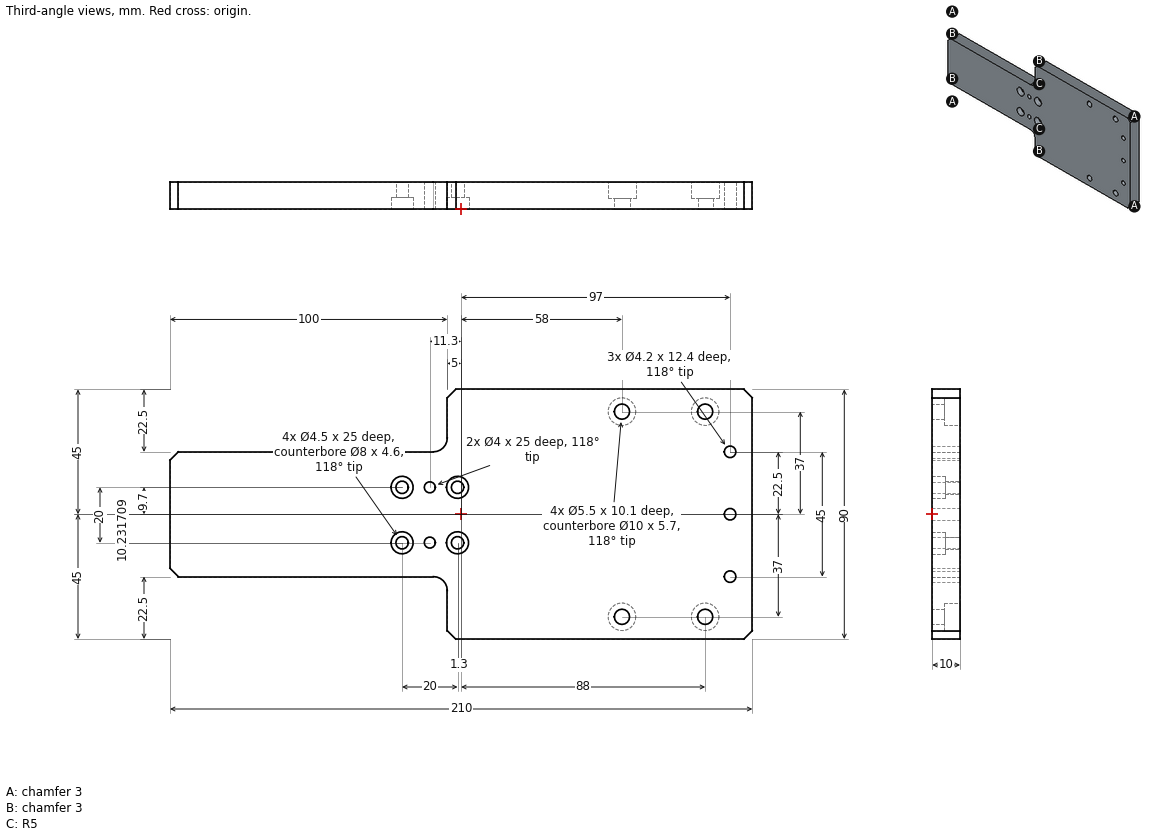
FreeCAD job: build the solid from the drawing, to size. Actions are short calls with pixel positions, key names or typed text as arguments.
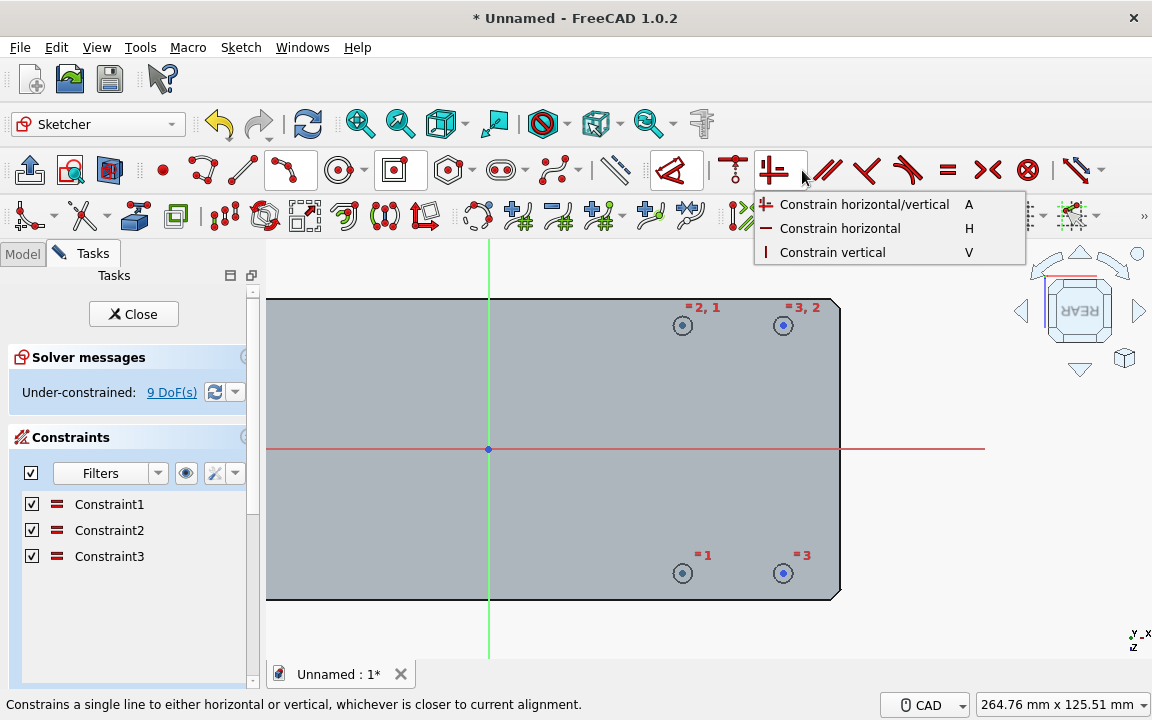
click(890, 252)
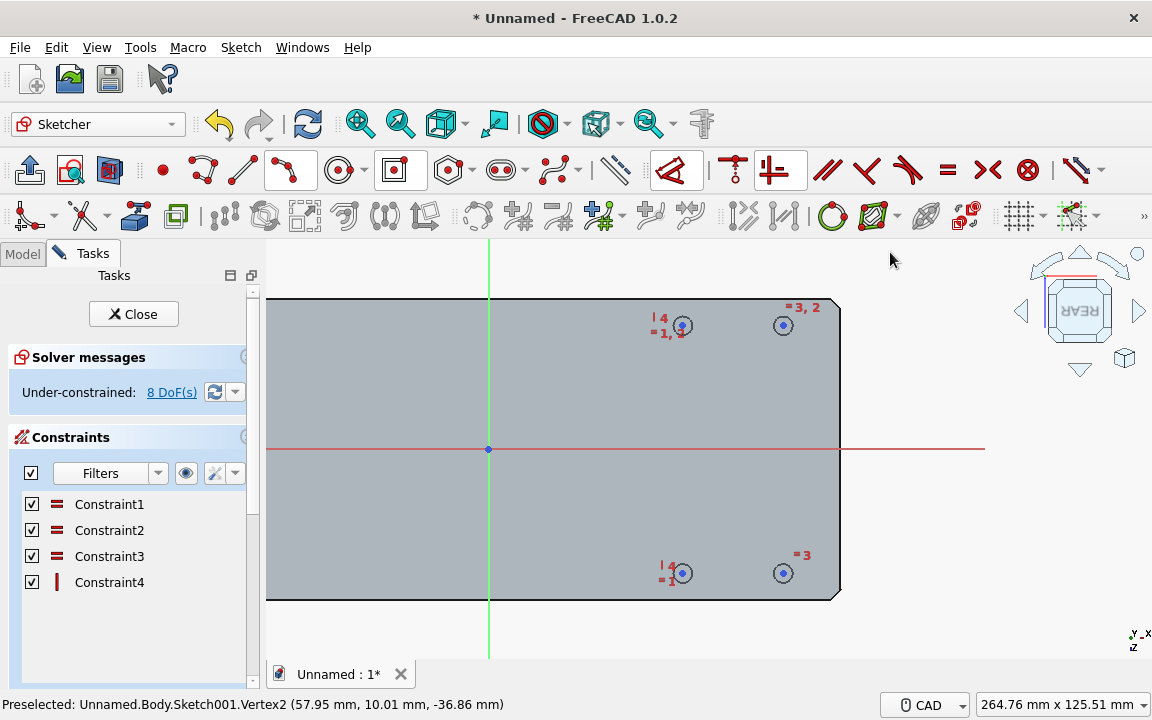
click(685, 328)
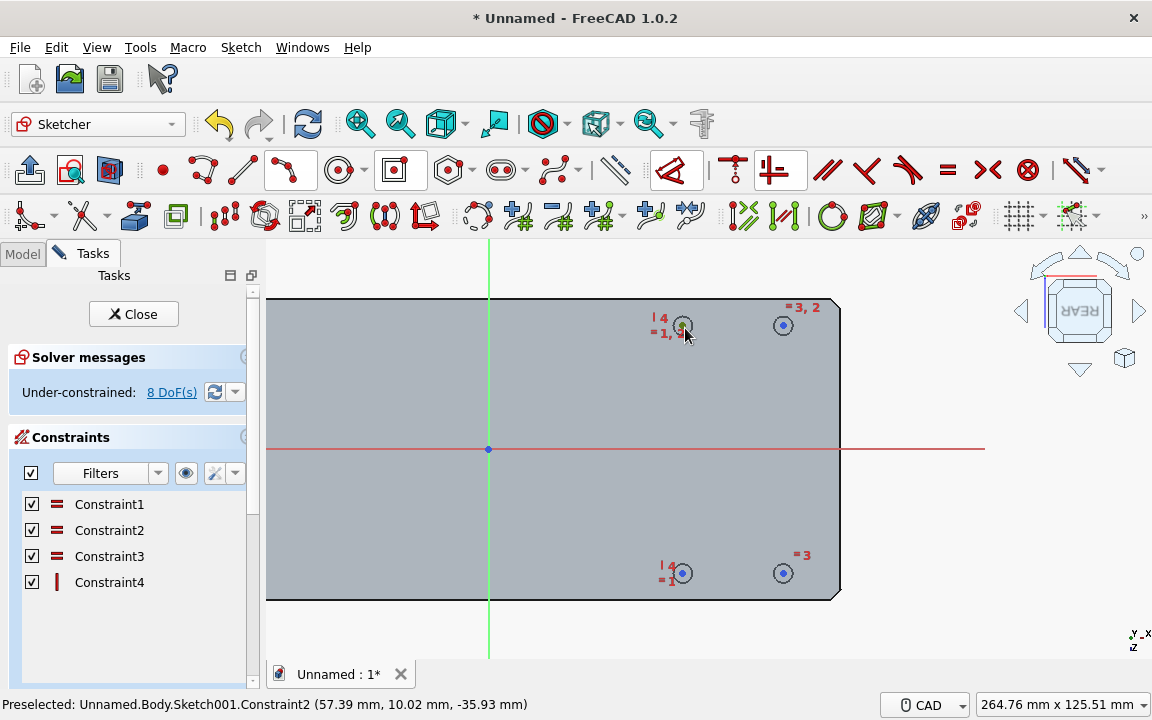
click(783, 326)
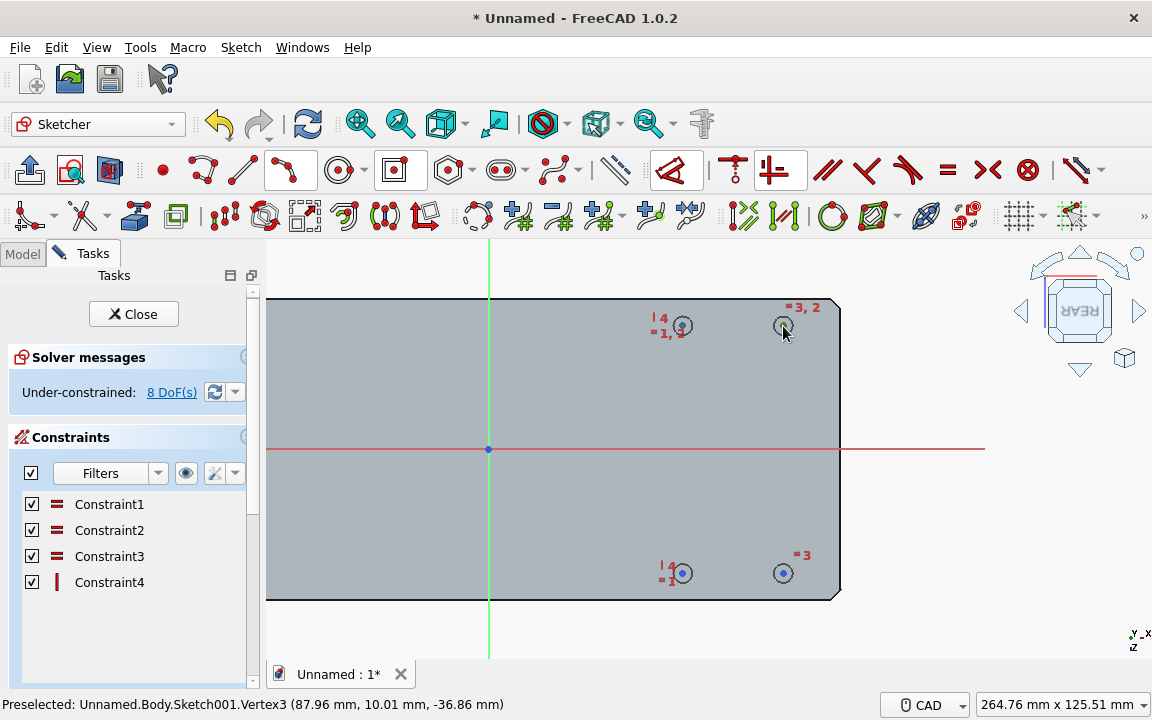
key(h)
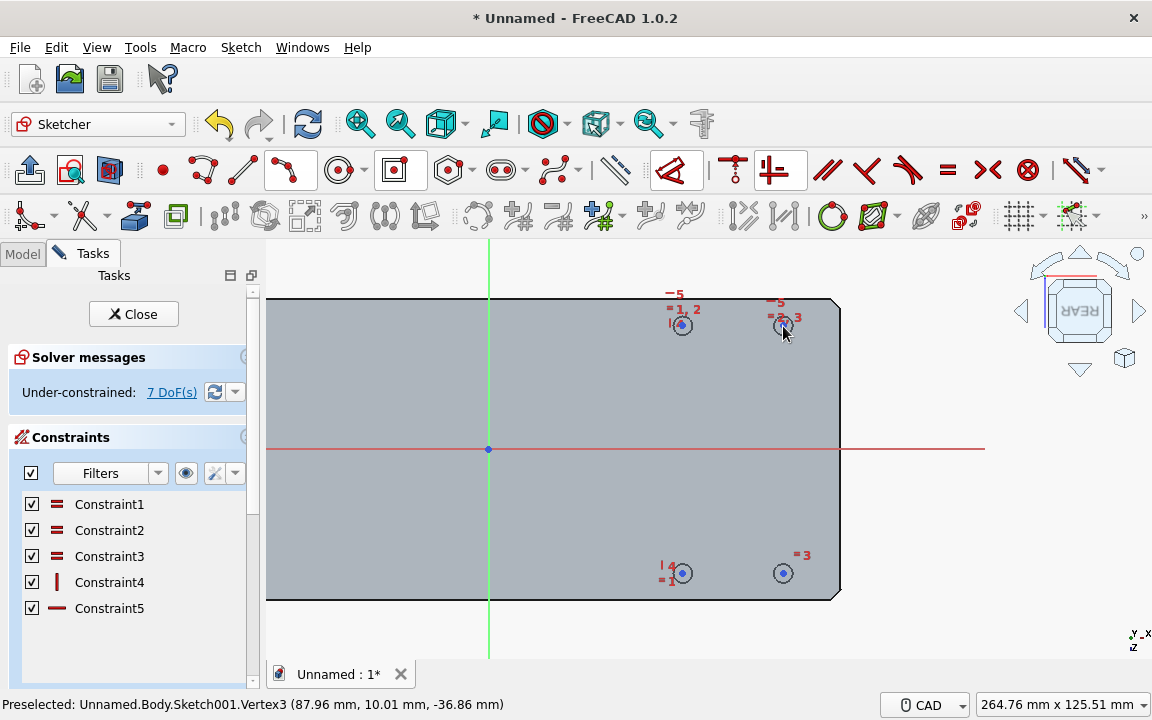
click(783, 326)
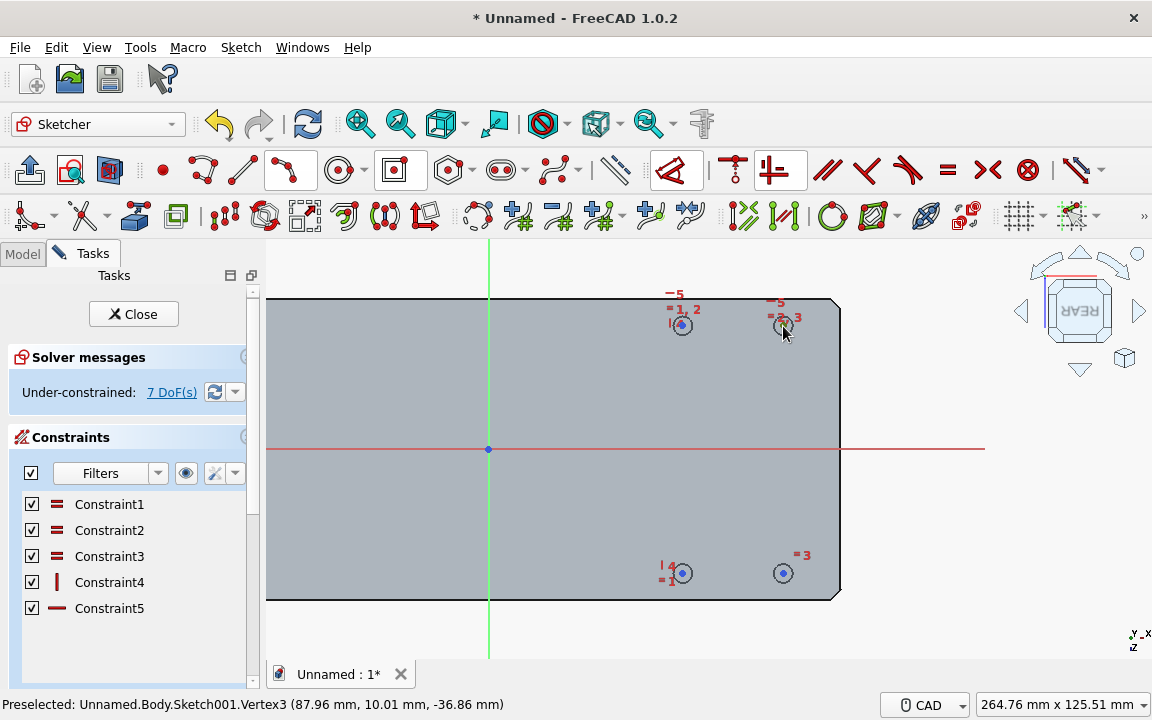
click(783, 574)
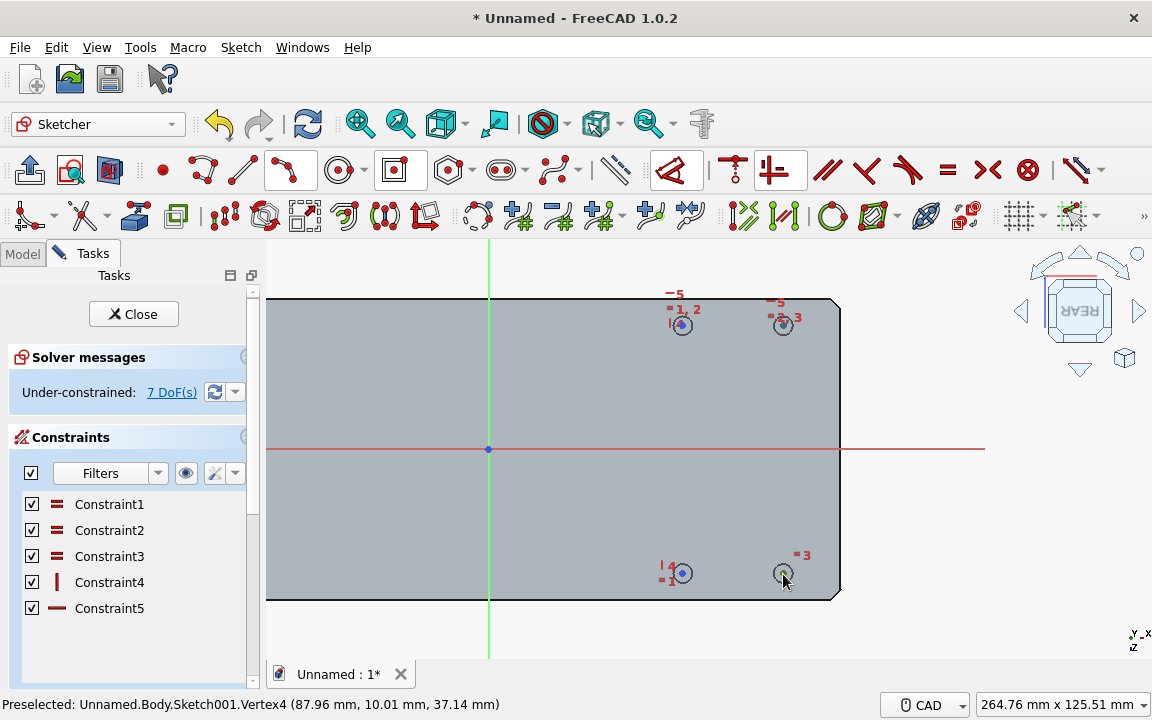
click(802, 170)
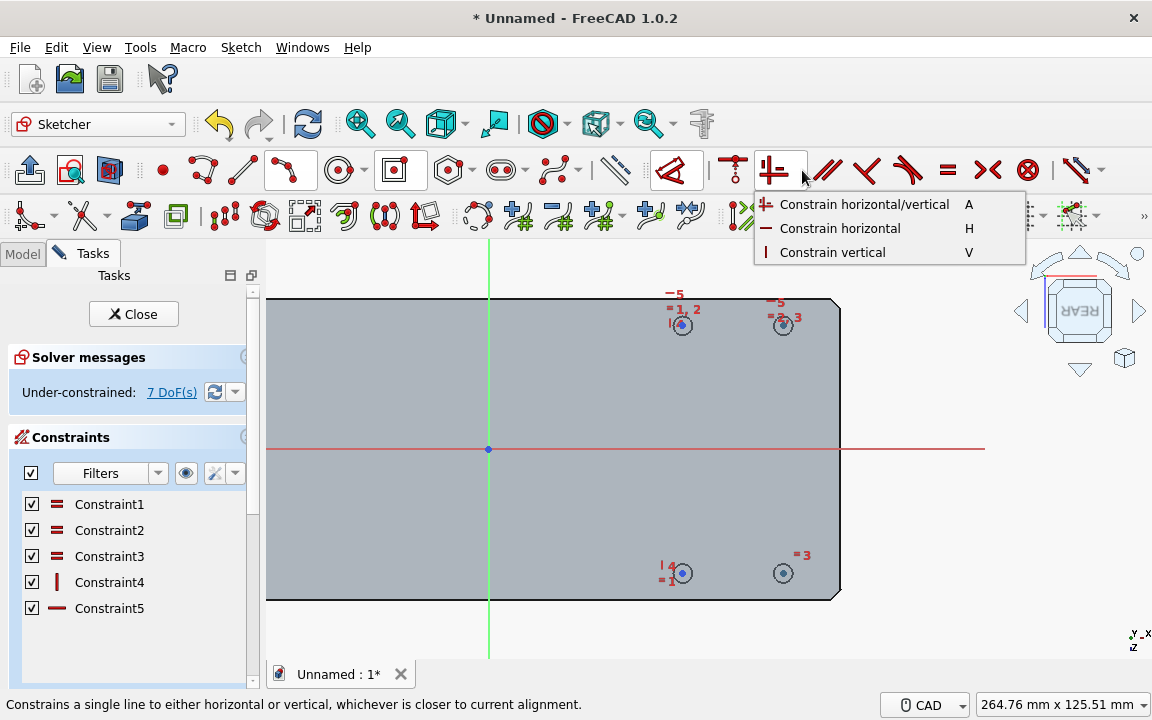
click(890, 252)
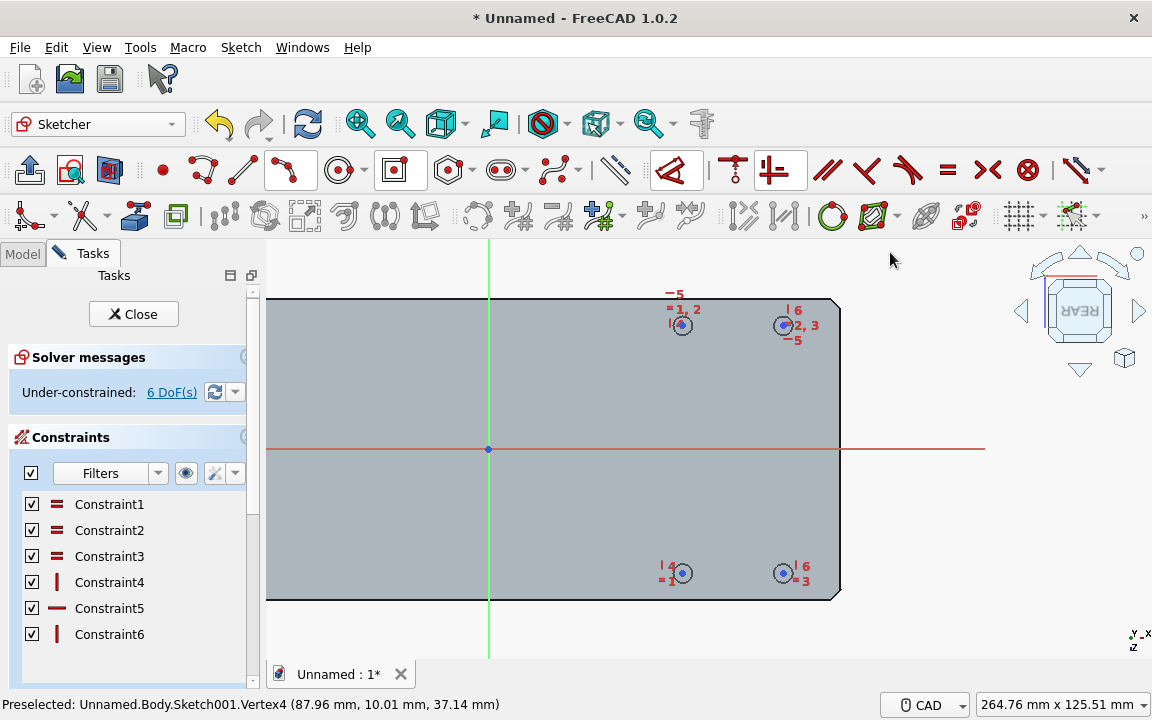
click(683, 574)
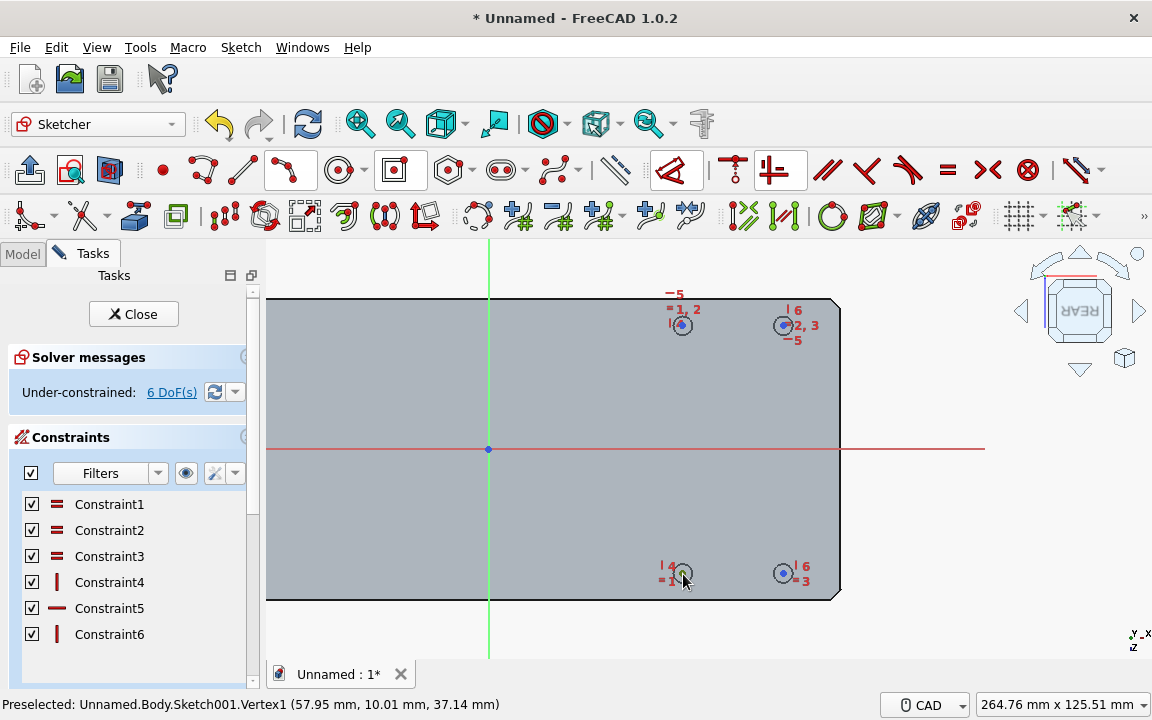
click(783, 574)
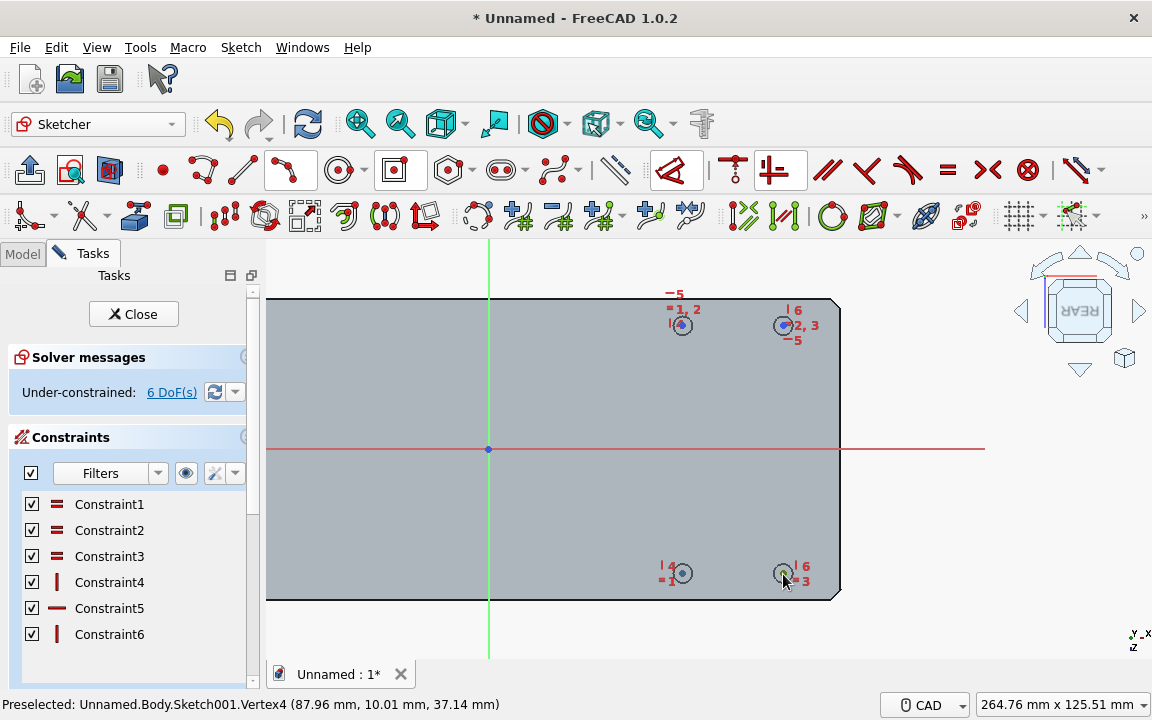
click(802, 170)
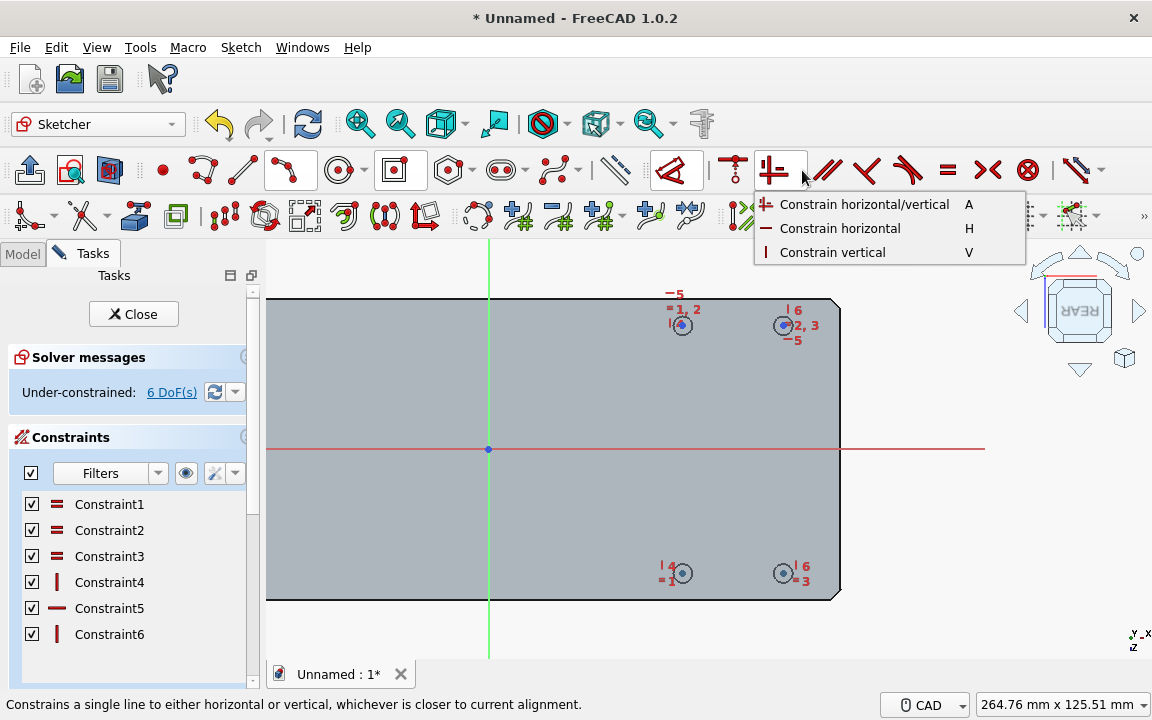
click(890, 228)